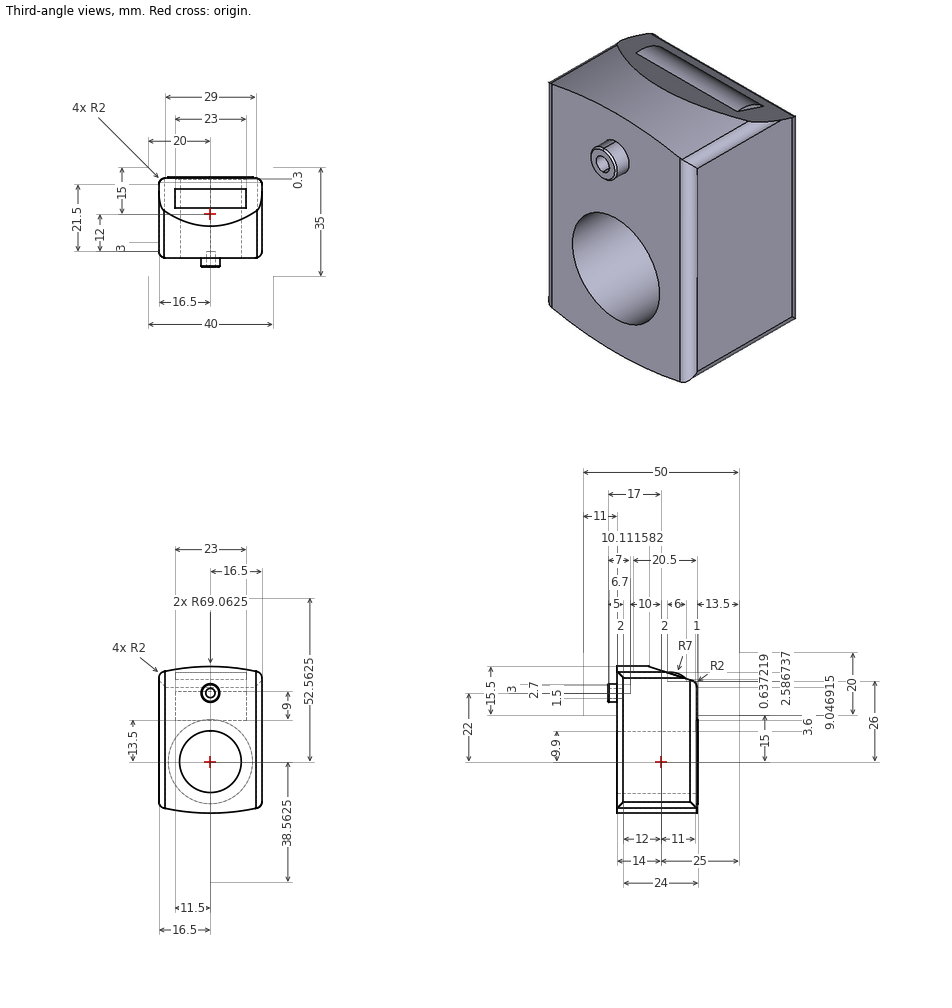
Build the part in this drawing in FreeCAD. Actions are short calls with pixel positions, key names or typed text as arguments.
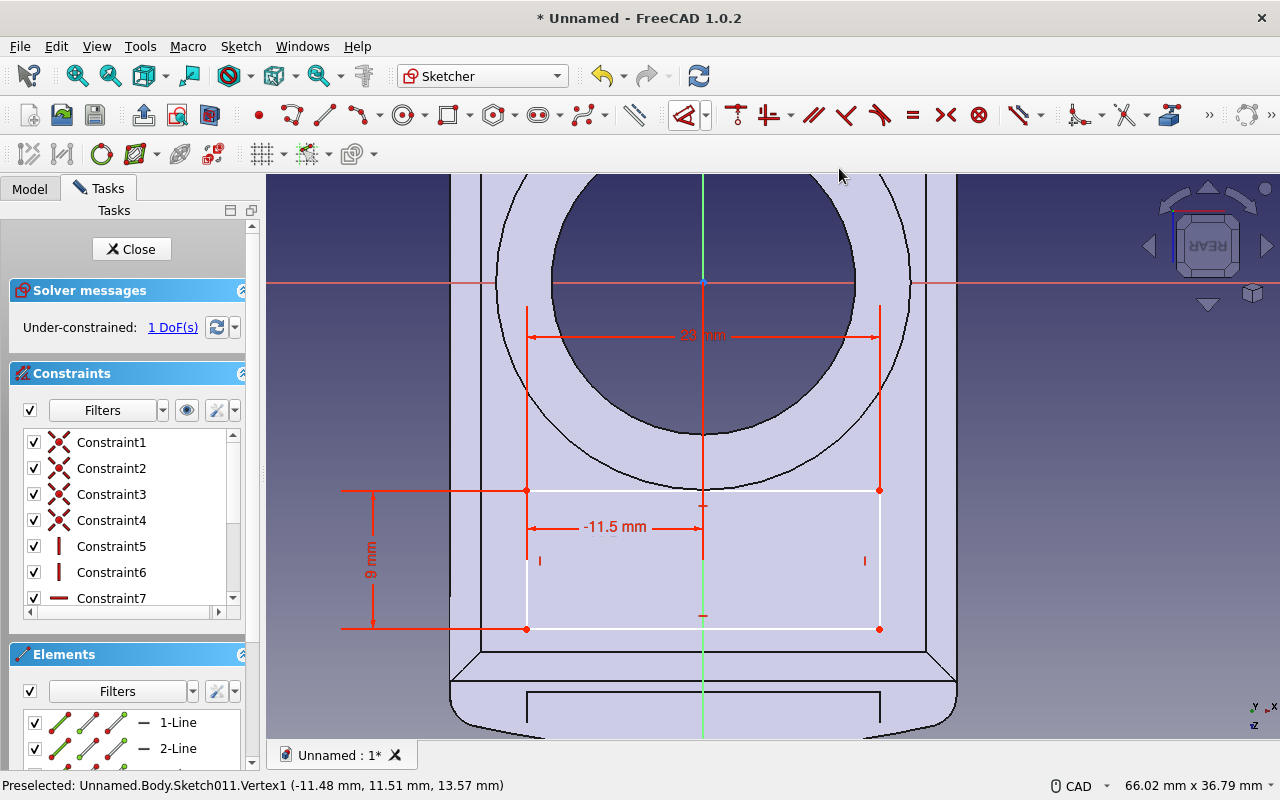
click(527, 491)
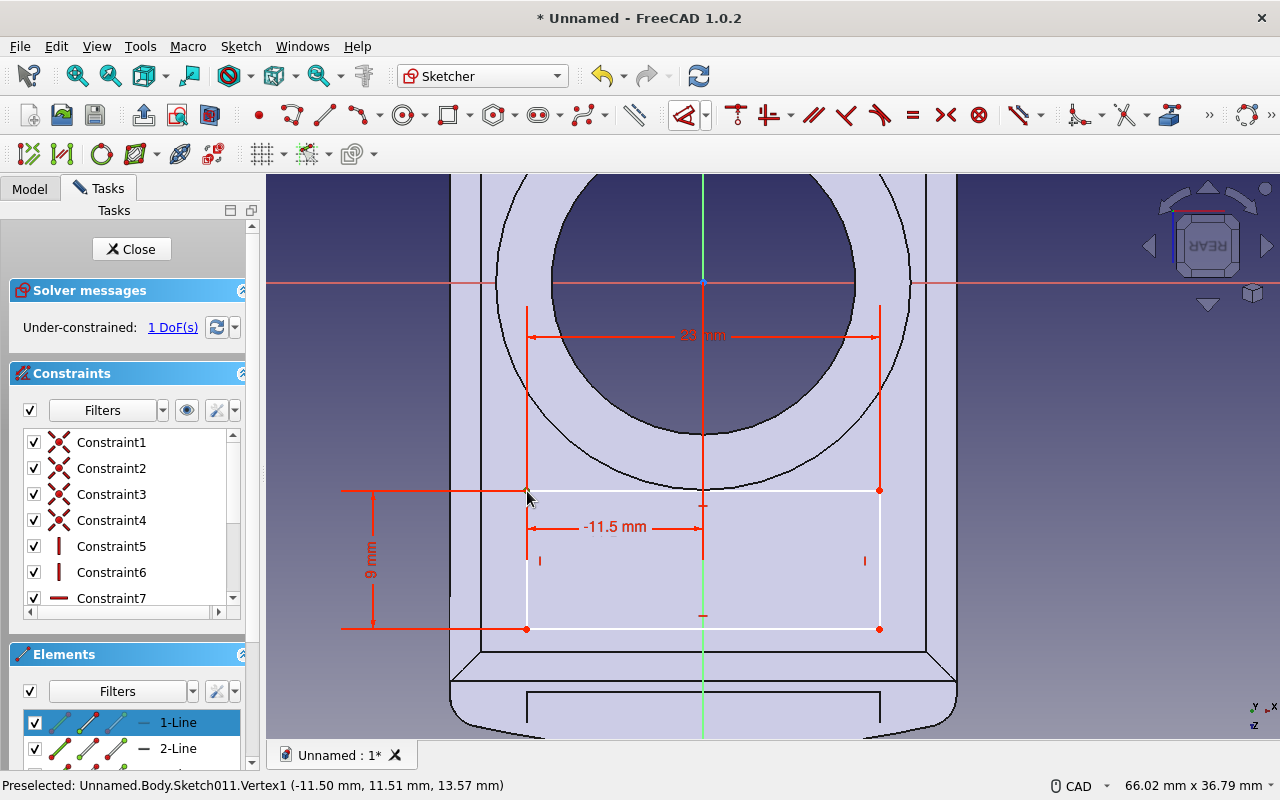
key(i)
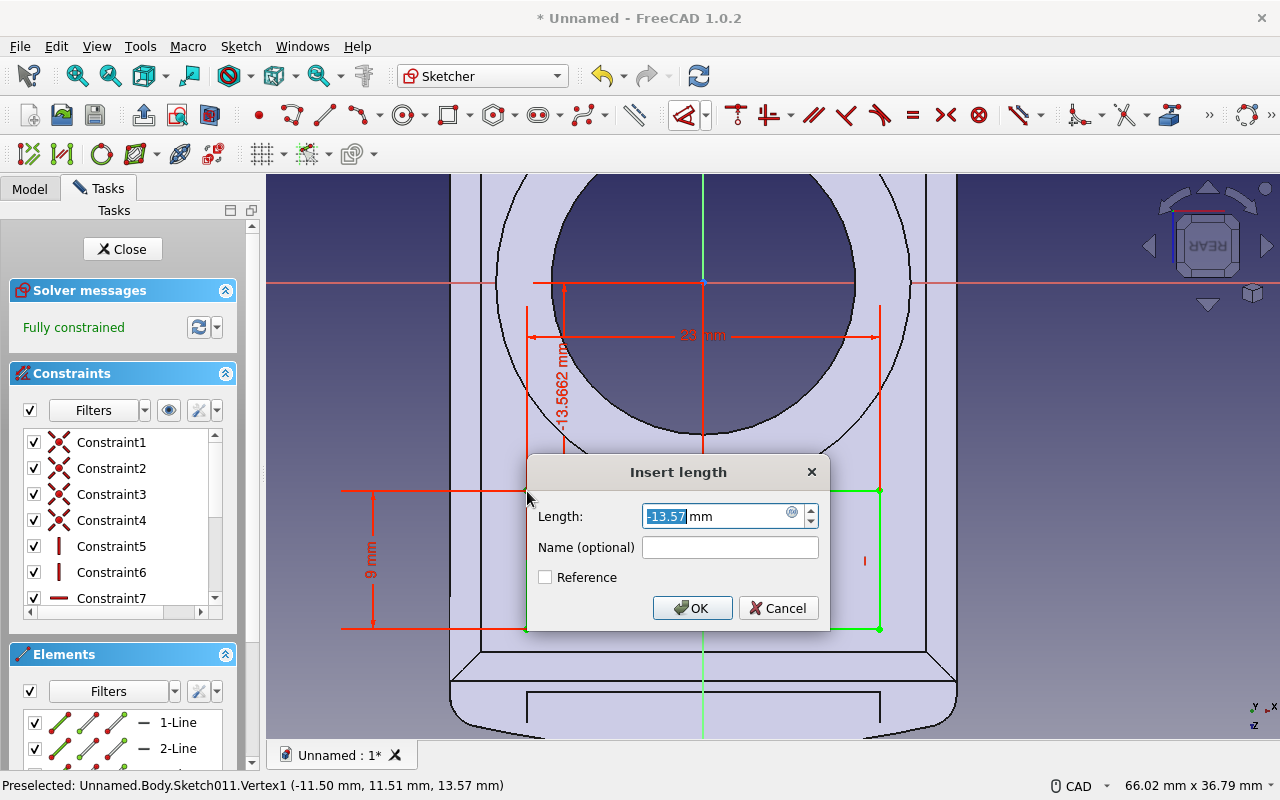
text(-13.5)
key(Return)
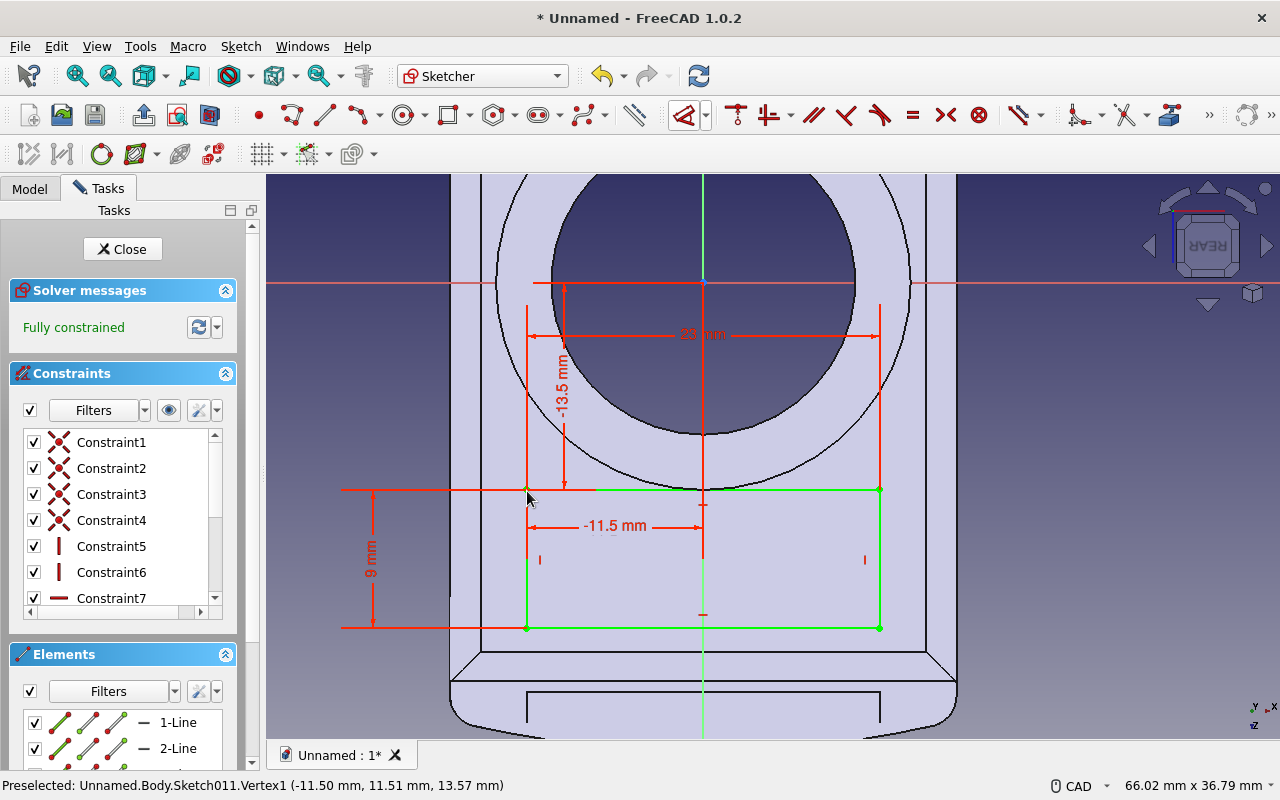
click(123, 249)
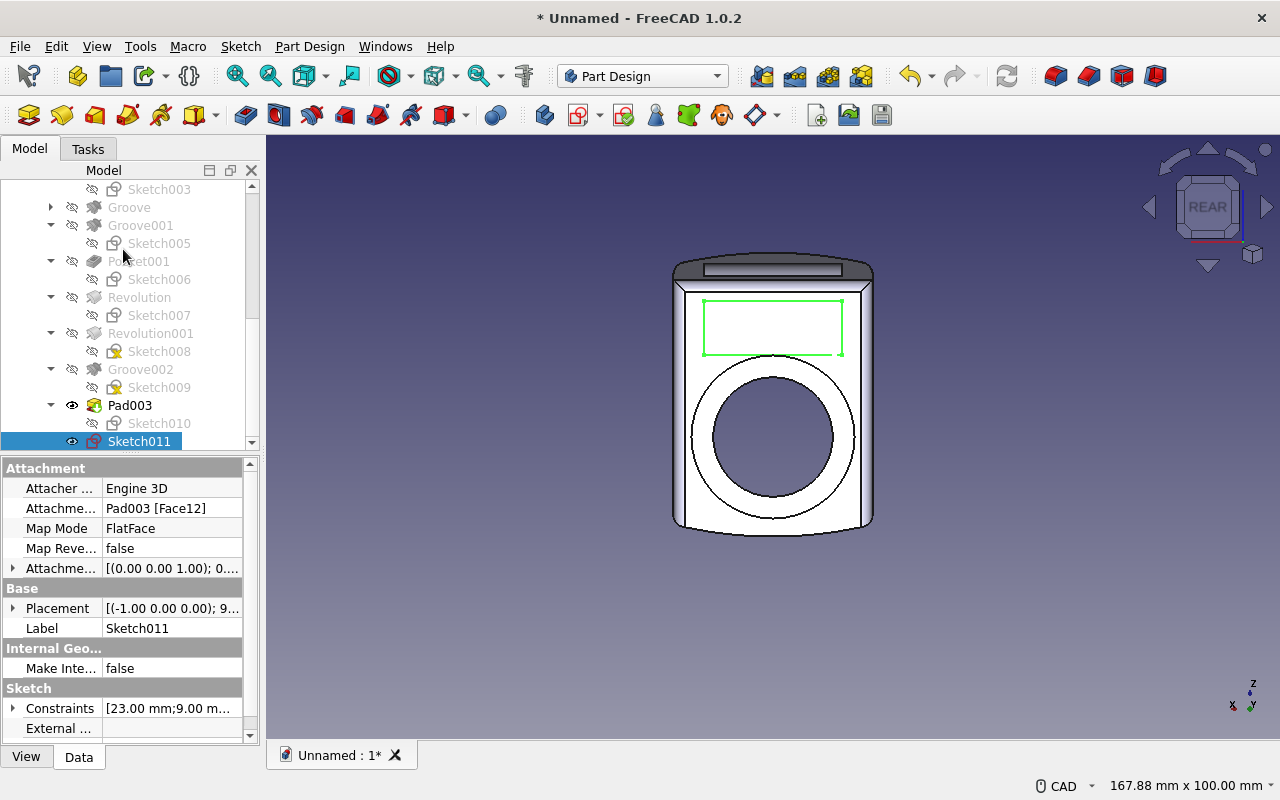
click(246, 116)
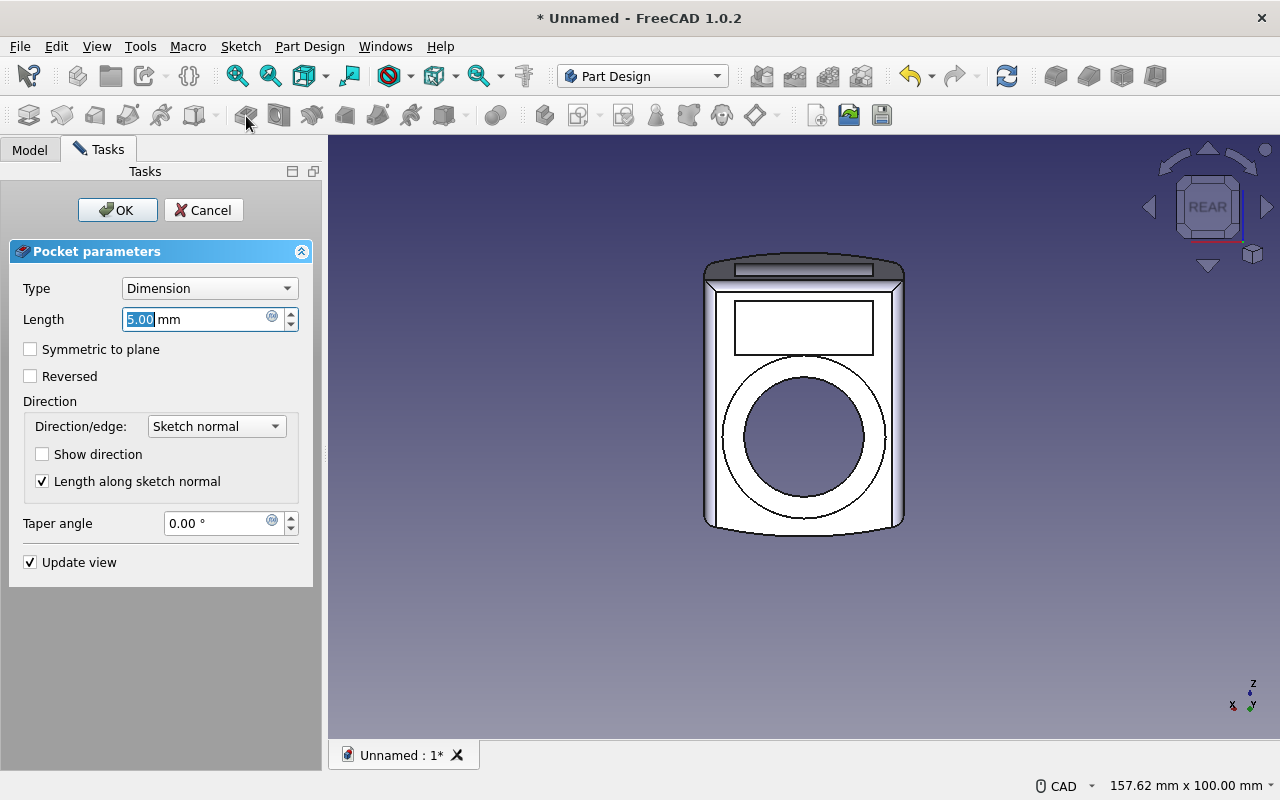
text(0.3)
key(Tab)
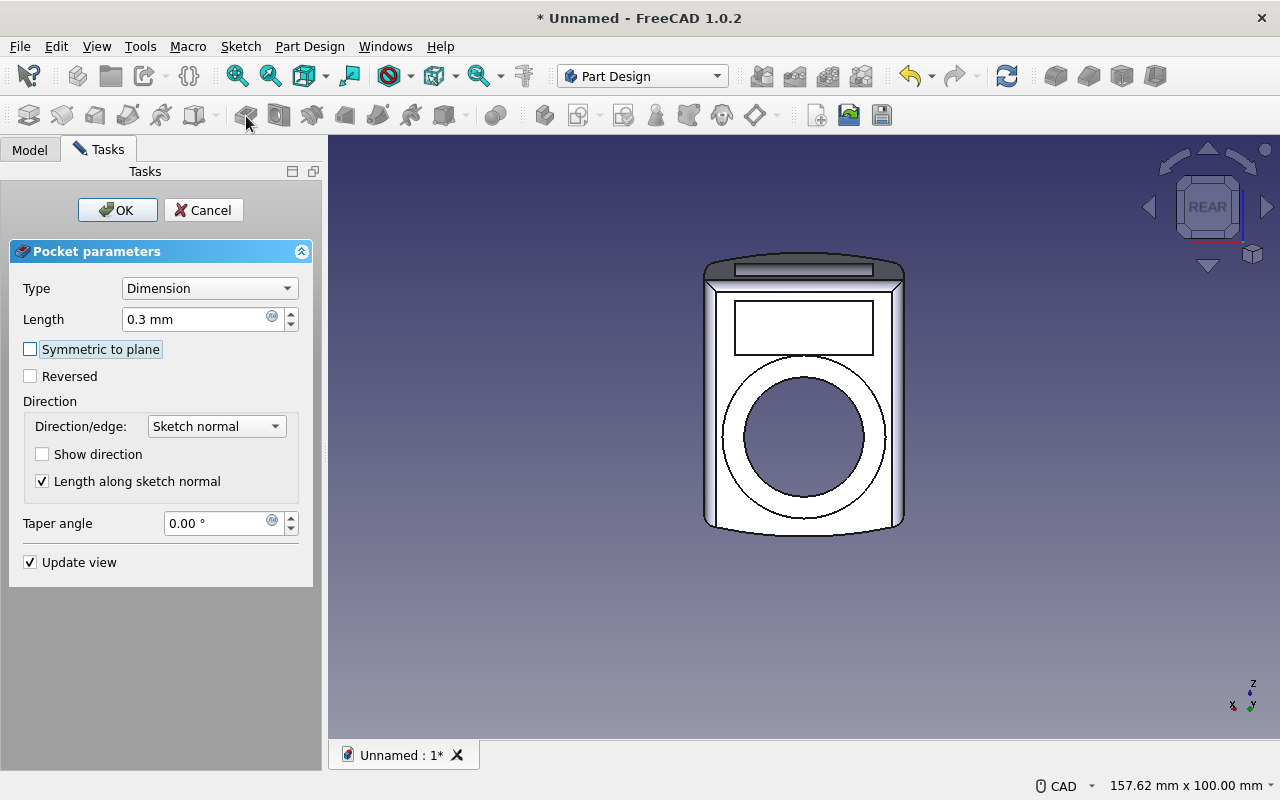
click(118, 210)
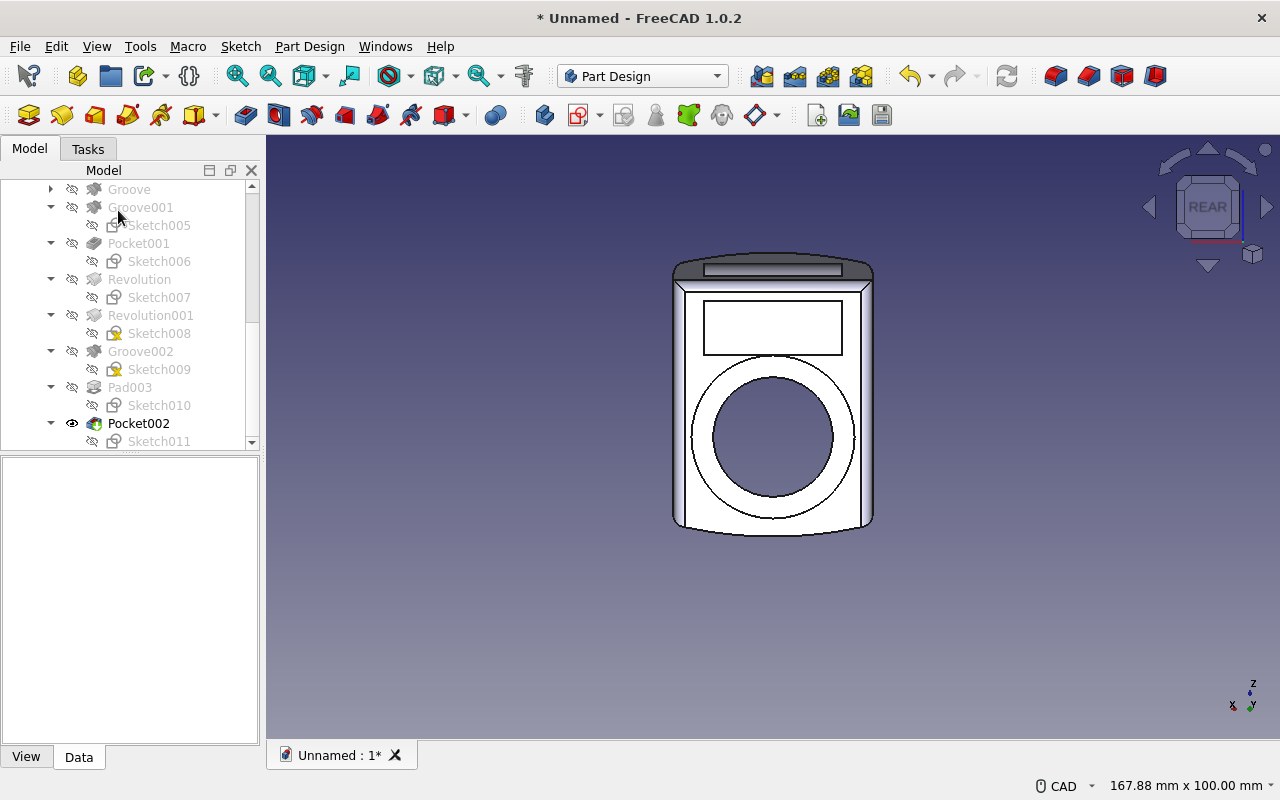
key(0)